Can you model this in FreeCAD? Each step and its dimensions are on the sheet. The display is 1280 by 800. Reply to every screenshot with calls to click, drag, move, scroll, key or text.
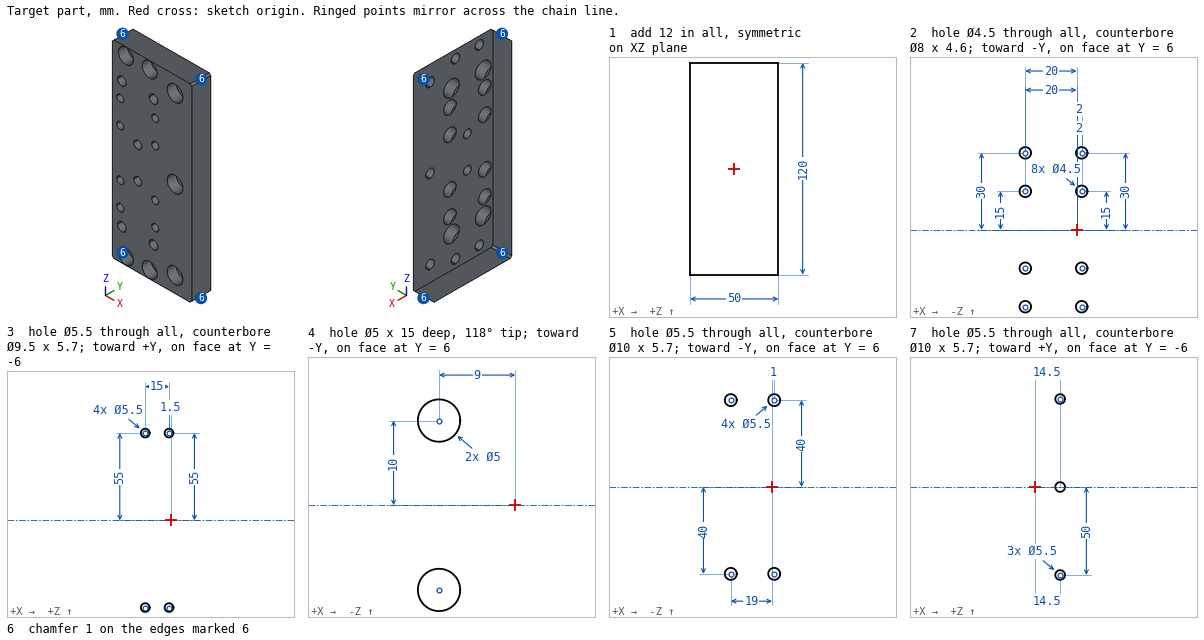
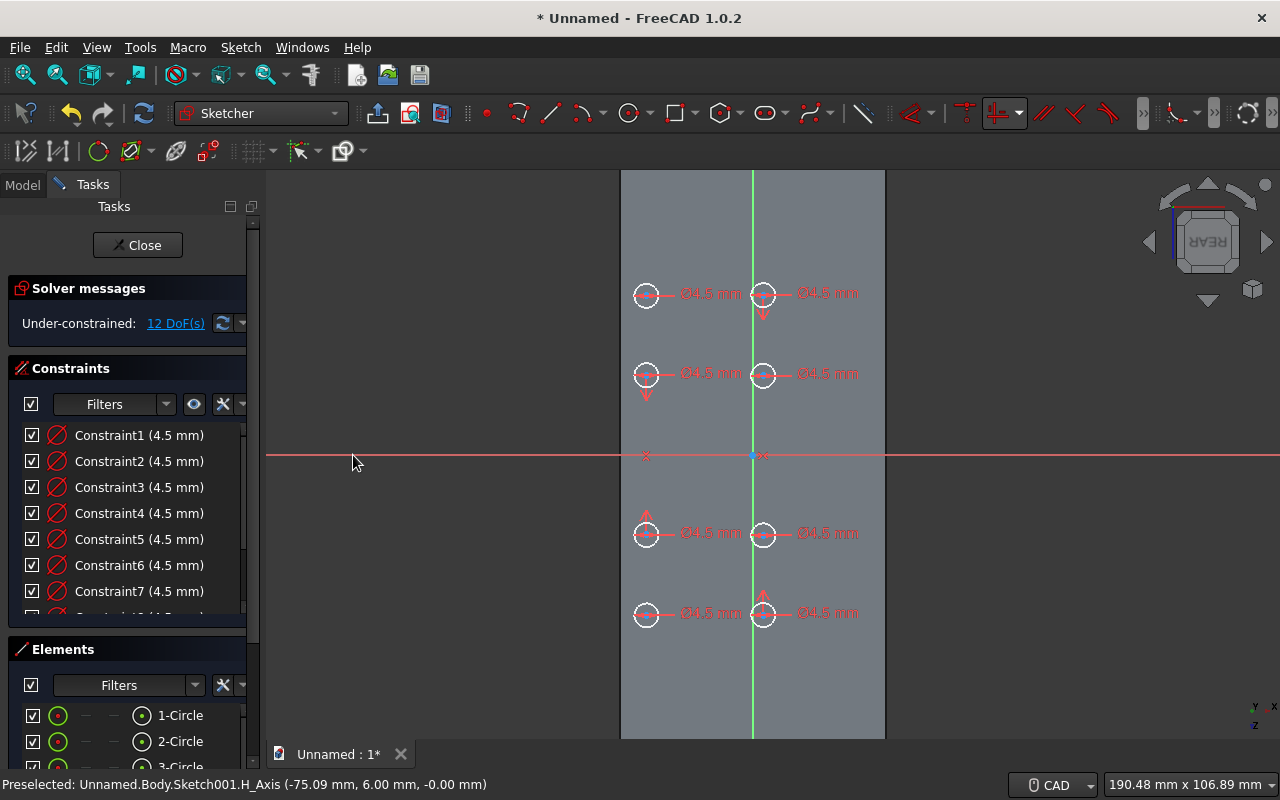
click(646, 296)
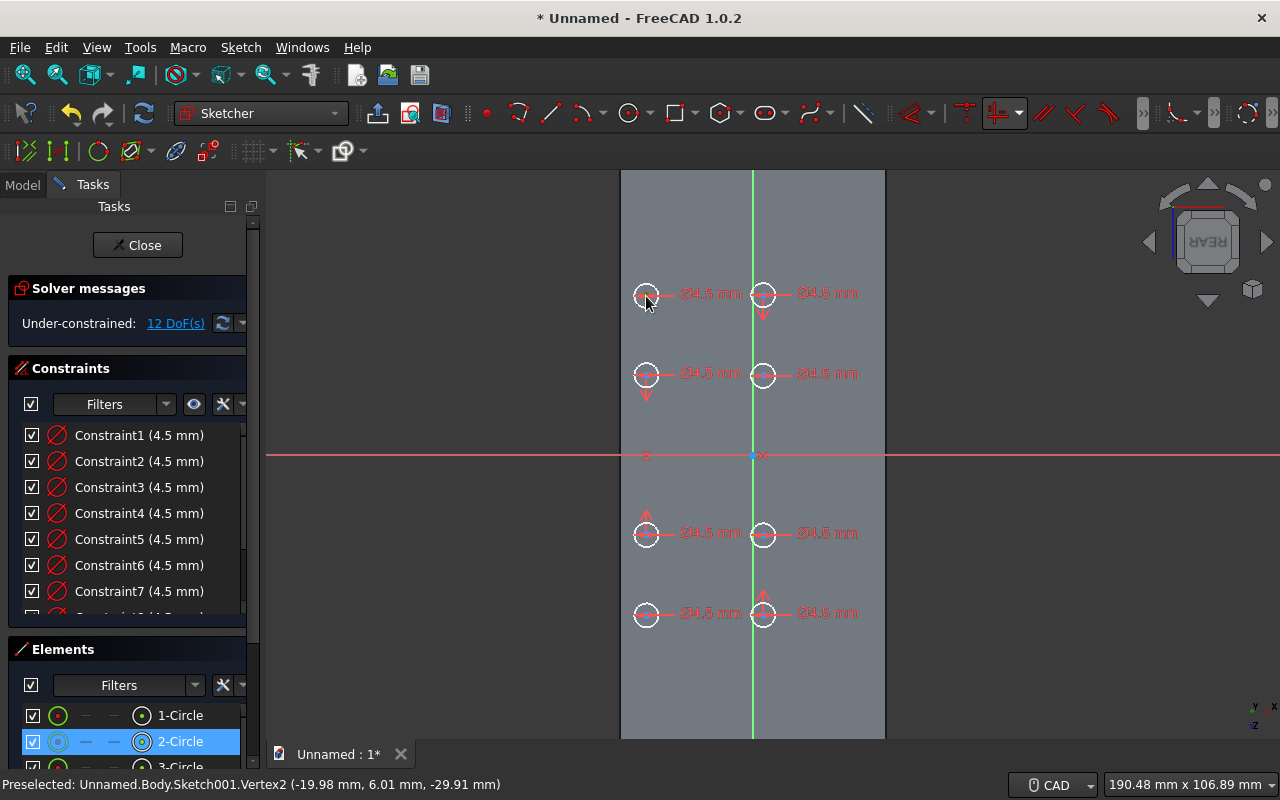
click(646, 615)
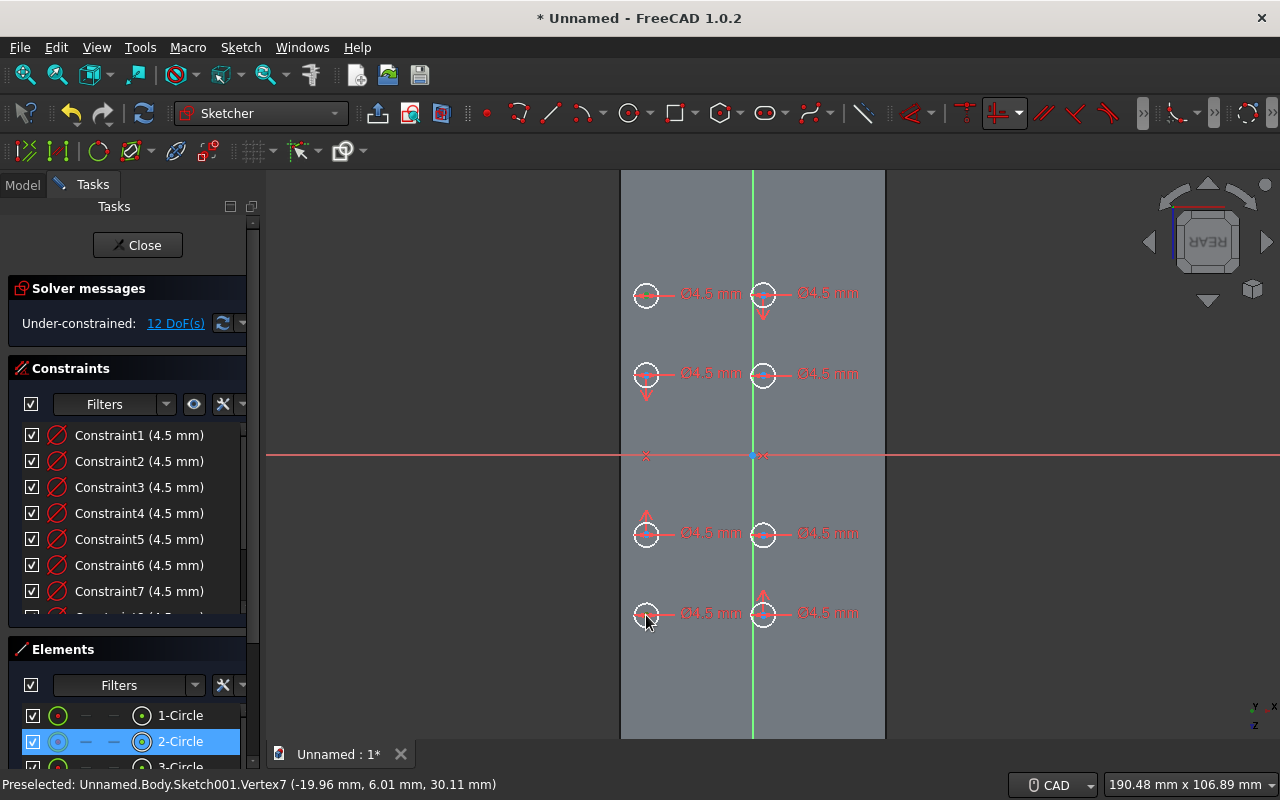
click(353, 455)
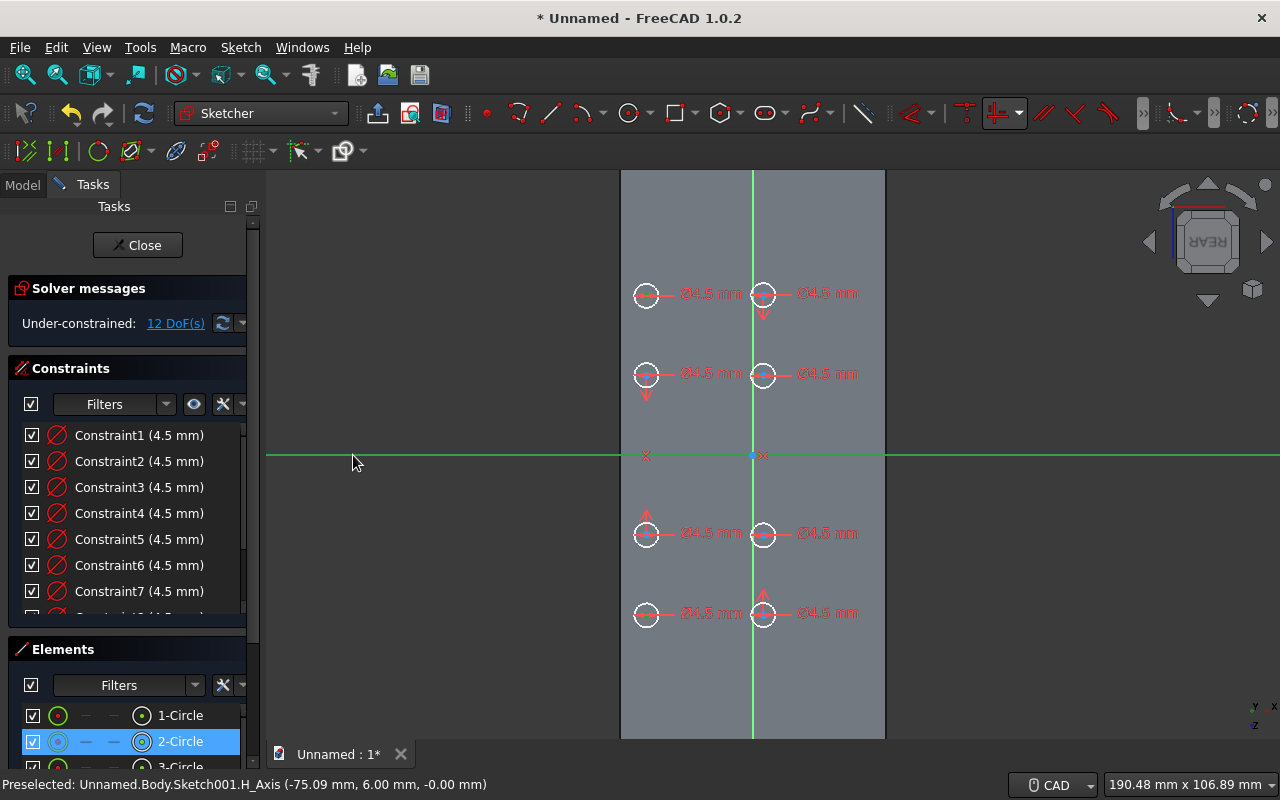
key(s)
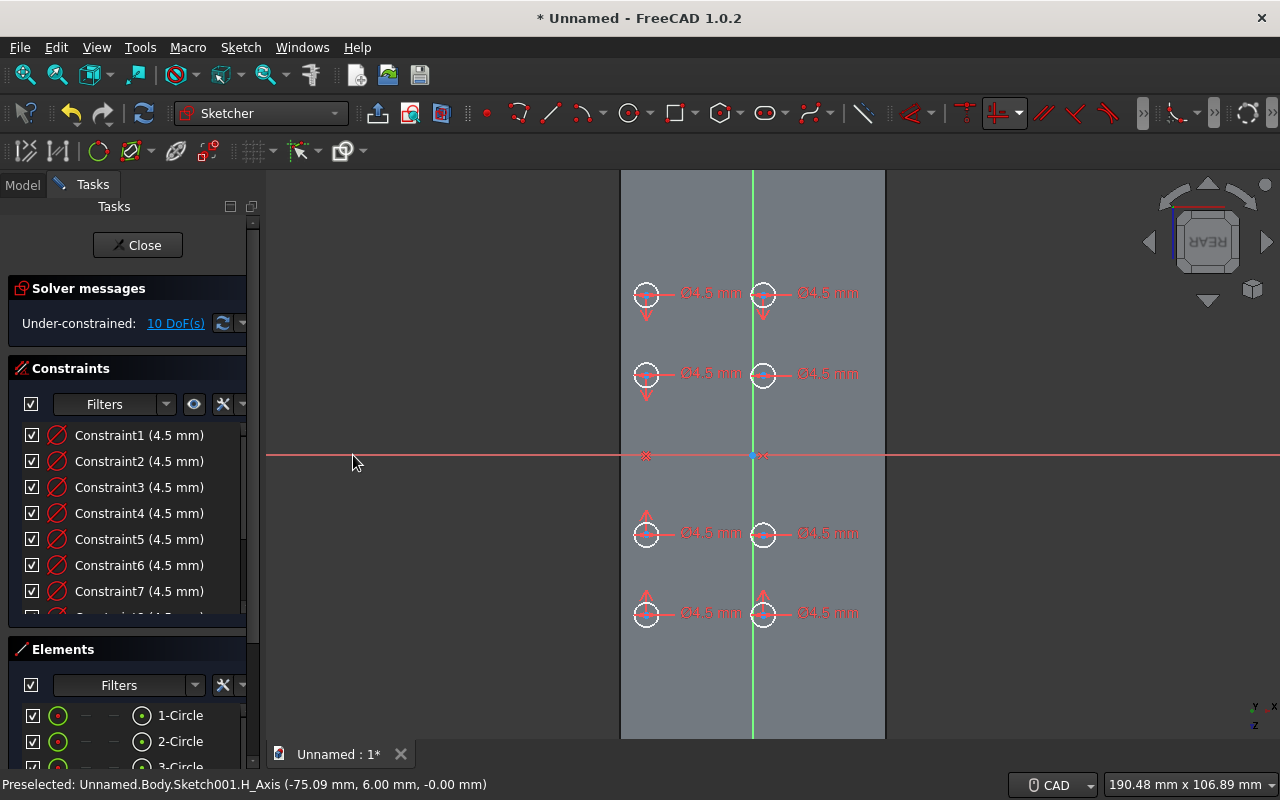
click(763, 376)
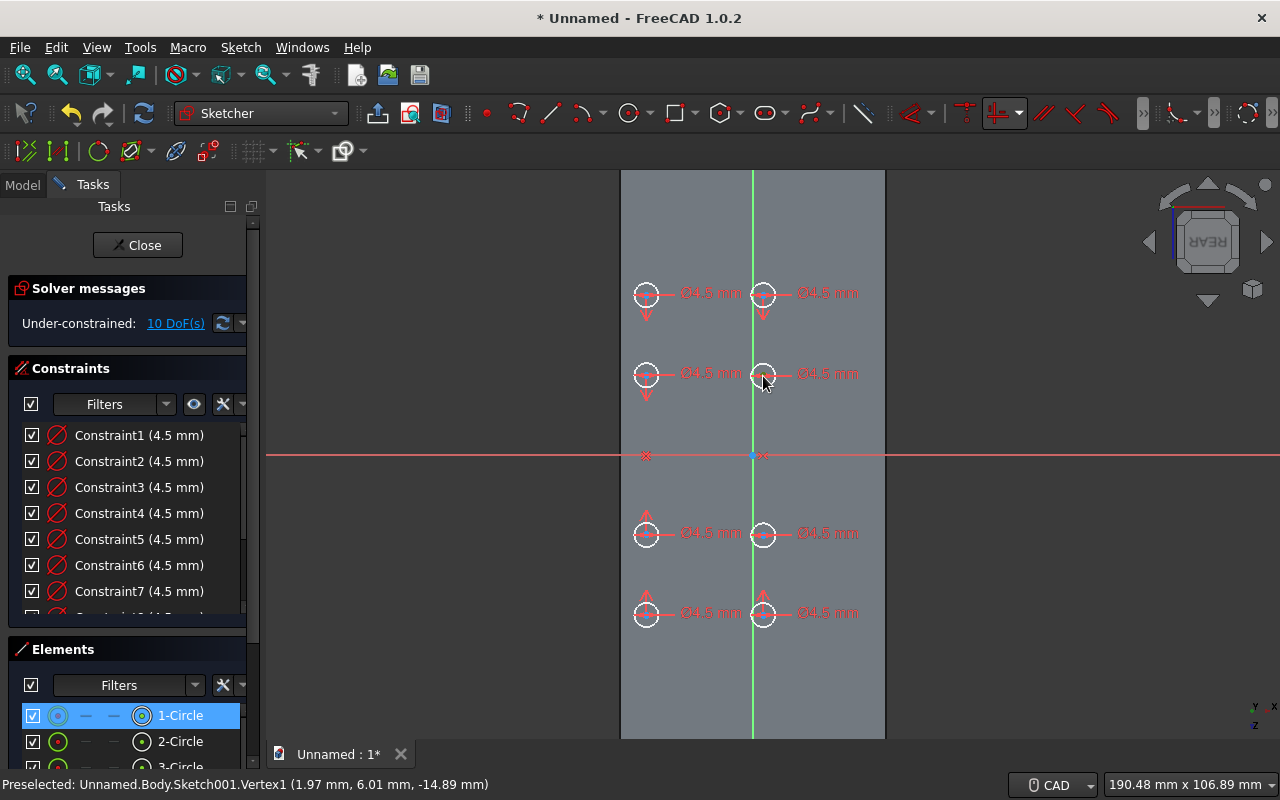
click(763, 535)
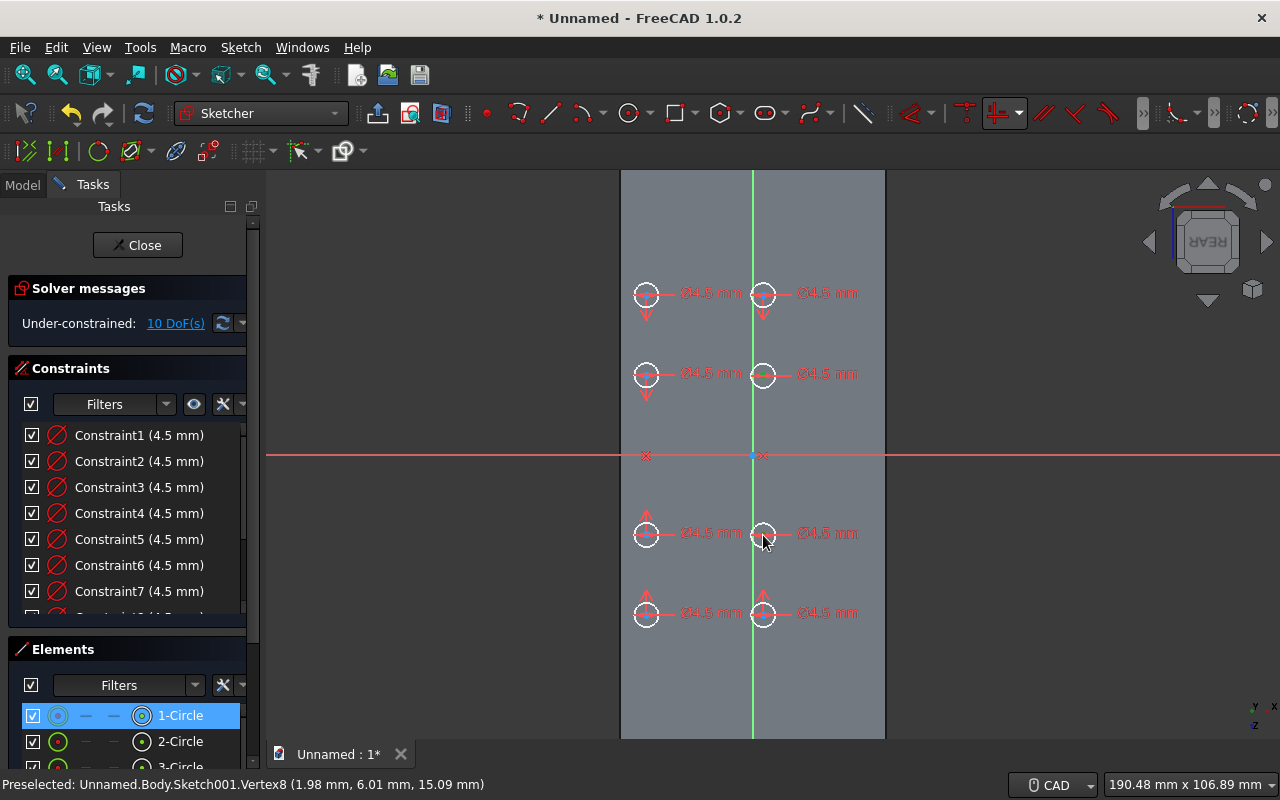
click(353, 455)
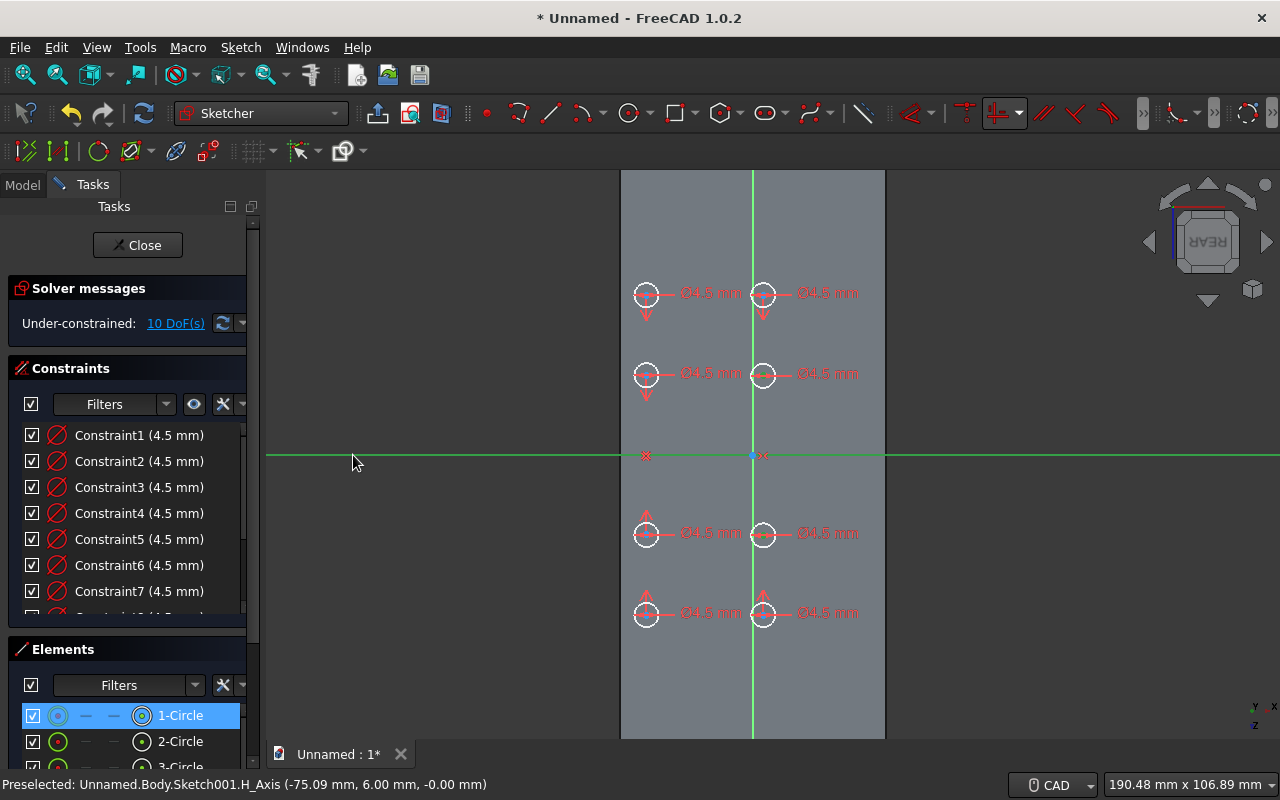
key(s)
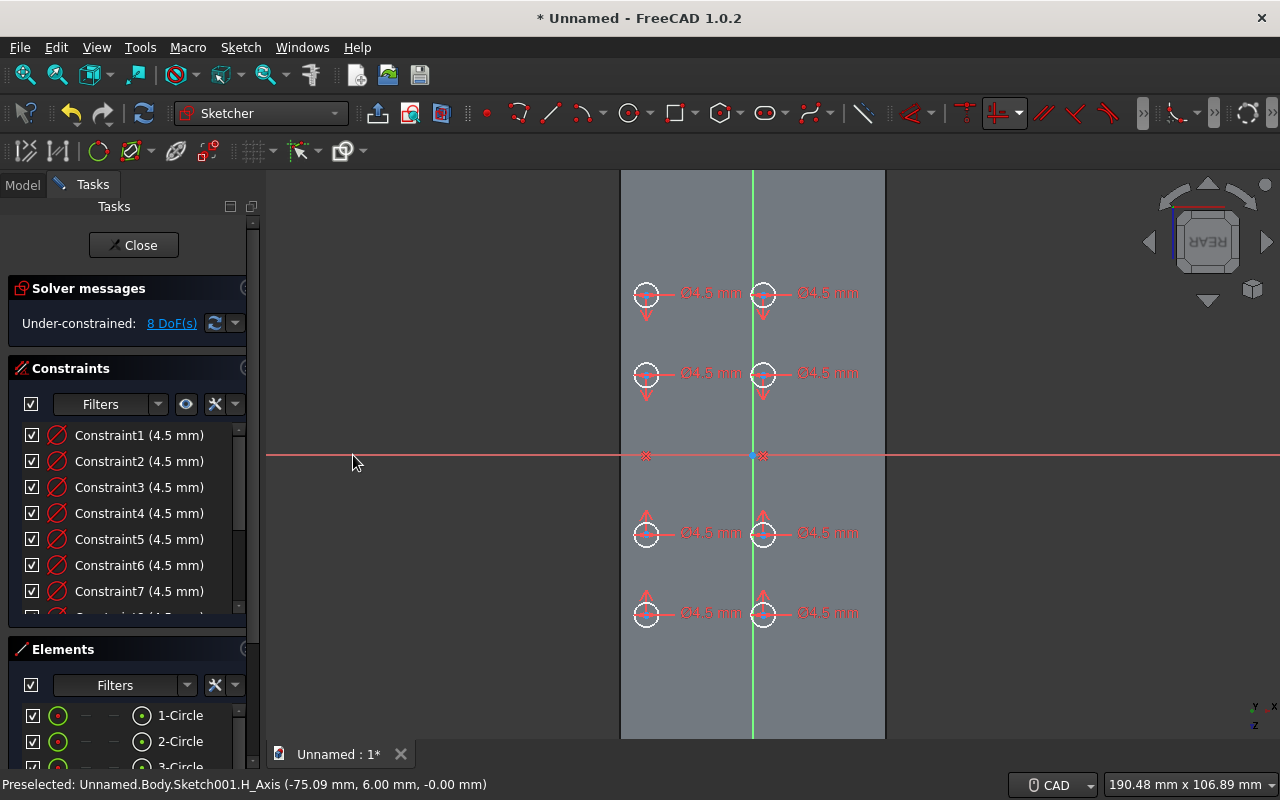
scroll(763, 375, up, 7)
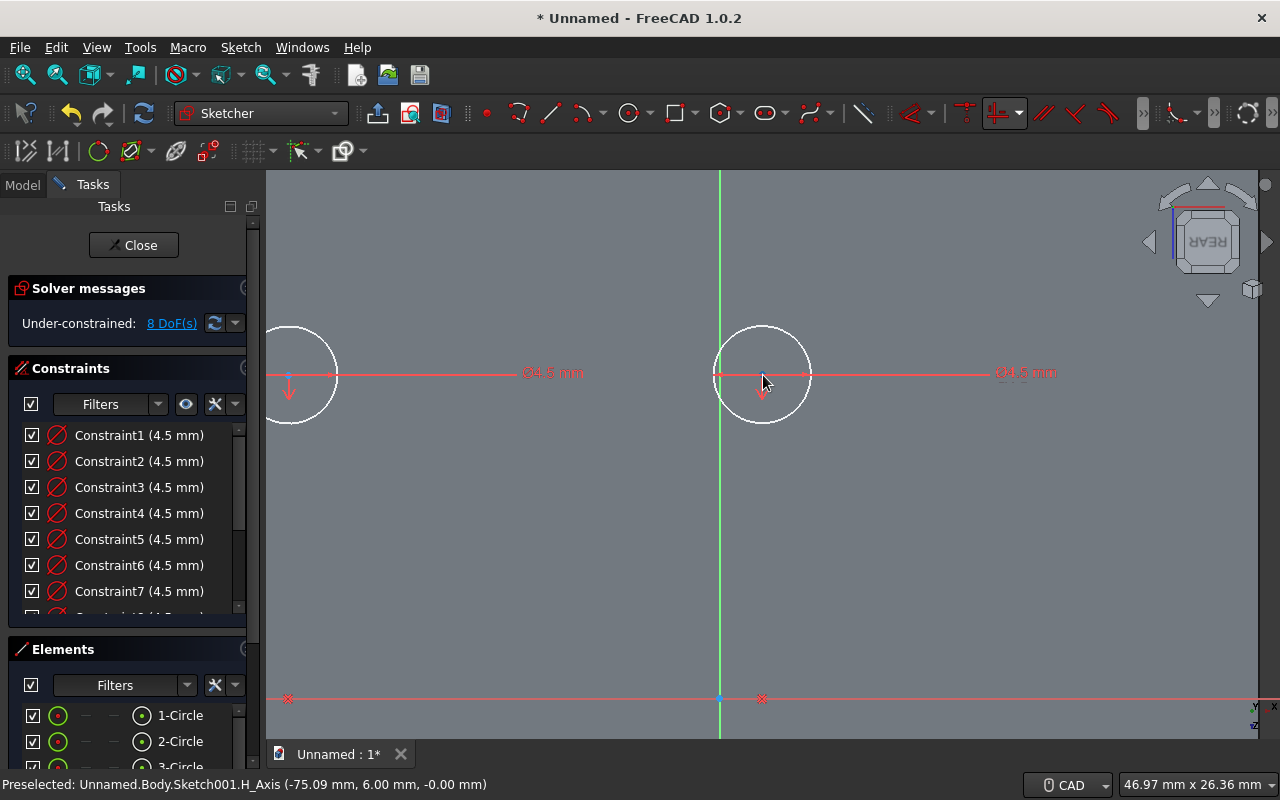
click(762, 375)